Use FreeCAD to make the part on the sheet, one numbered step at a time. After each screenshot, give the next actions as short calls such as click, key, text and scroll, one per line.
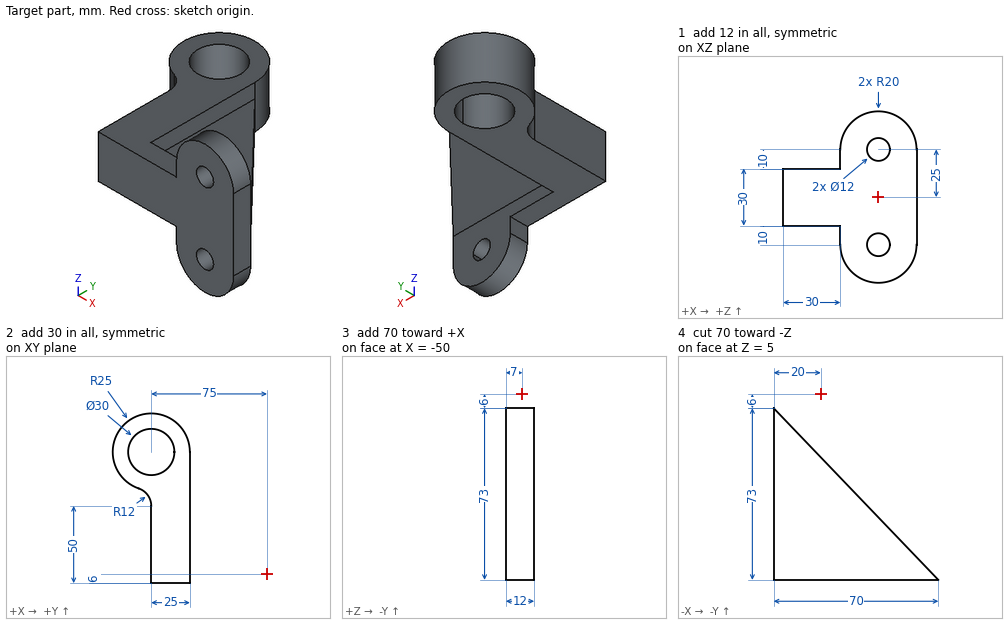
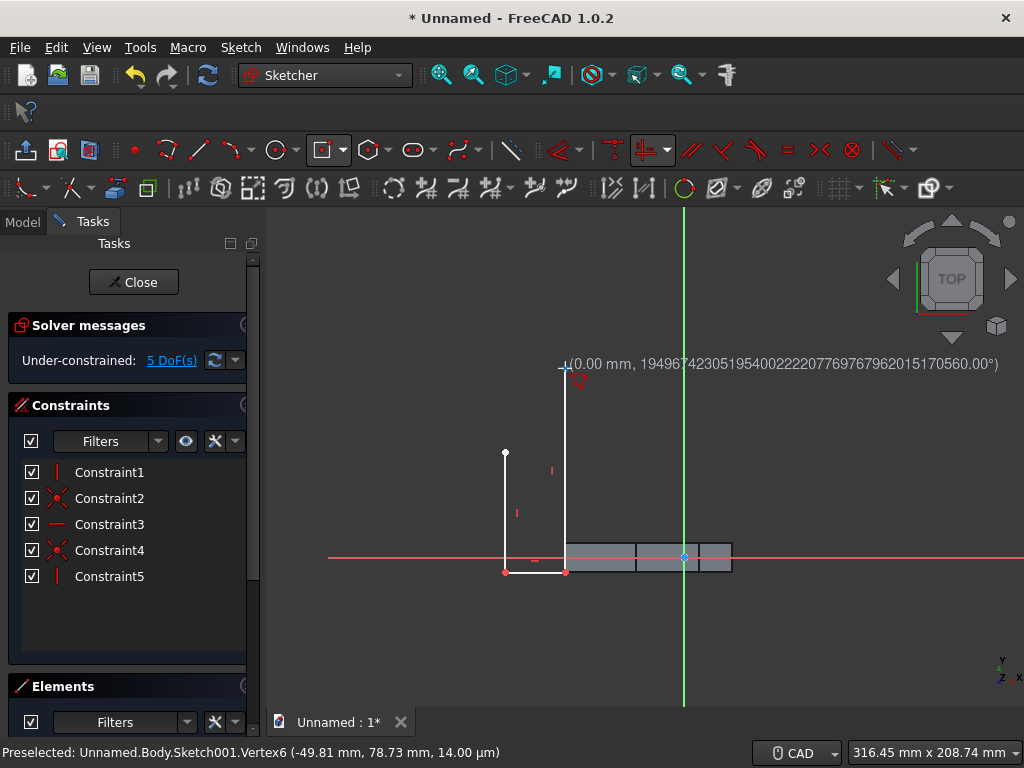
click(232, 150)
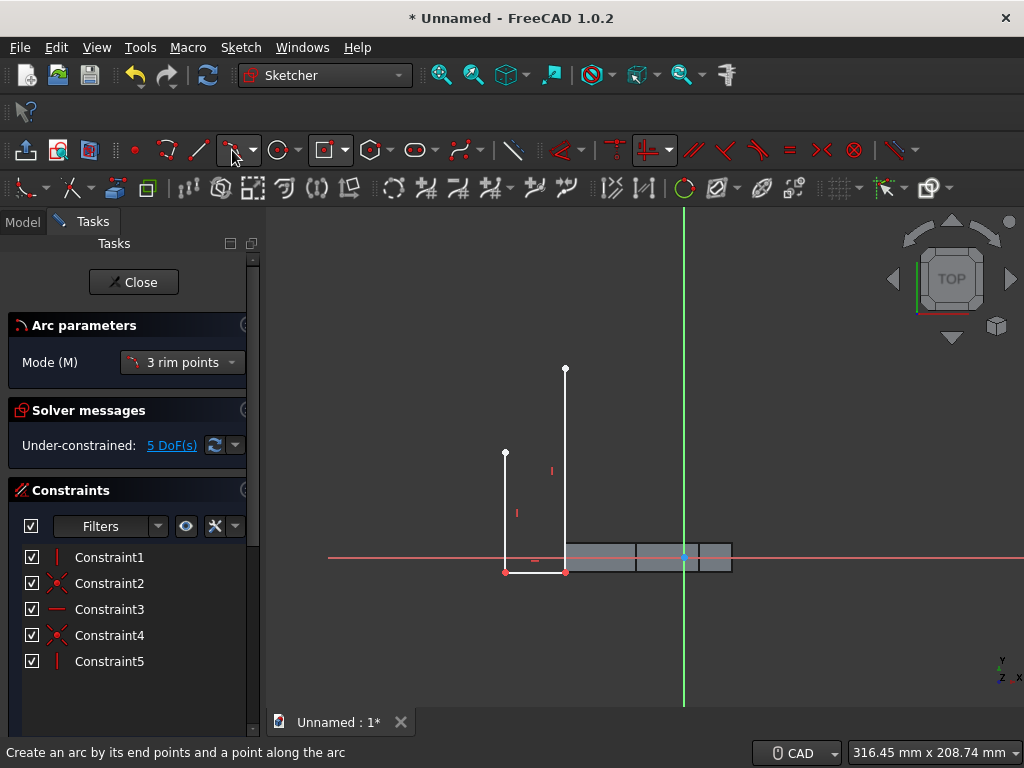
click(565, 369)
click(485, 425)
click(470, 320)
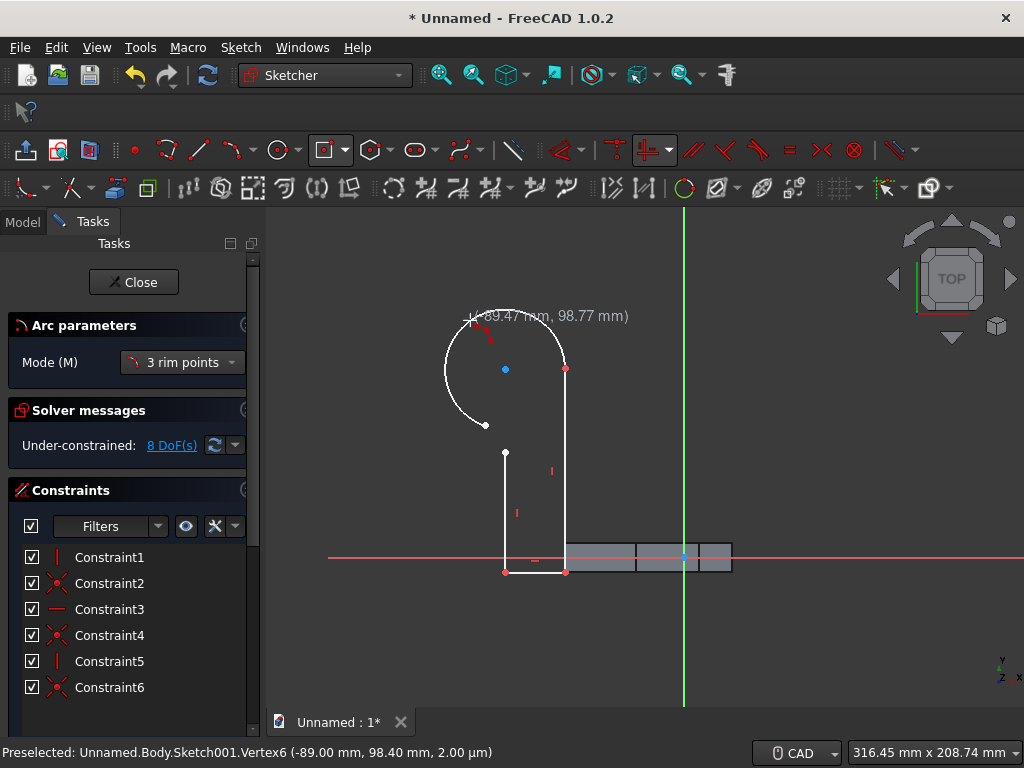
click(485, 426)
click(505, 453)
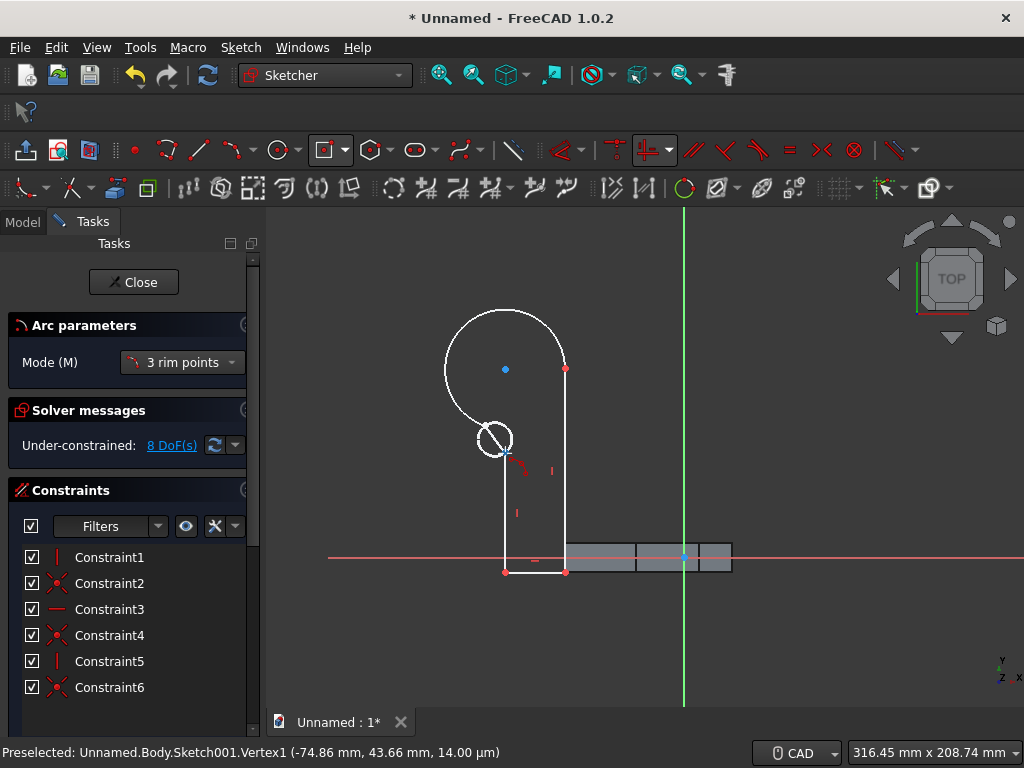
scroll(499, 435, up, 6)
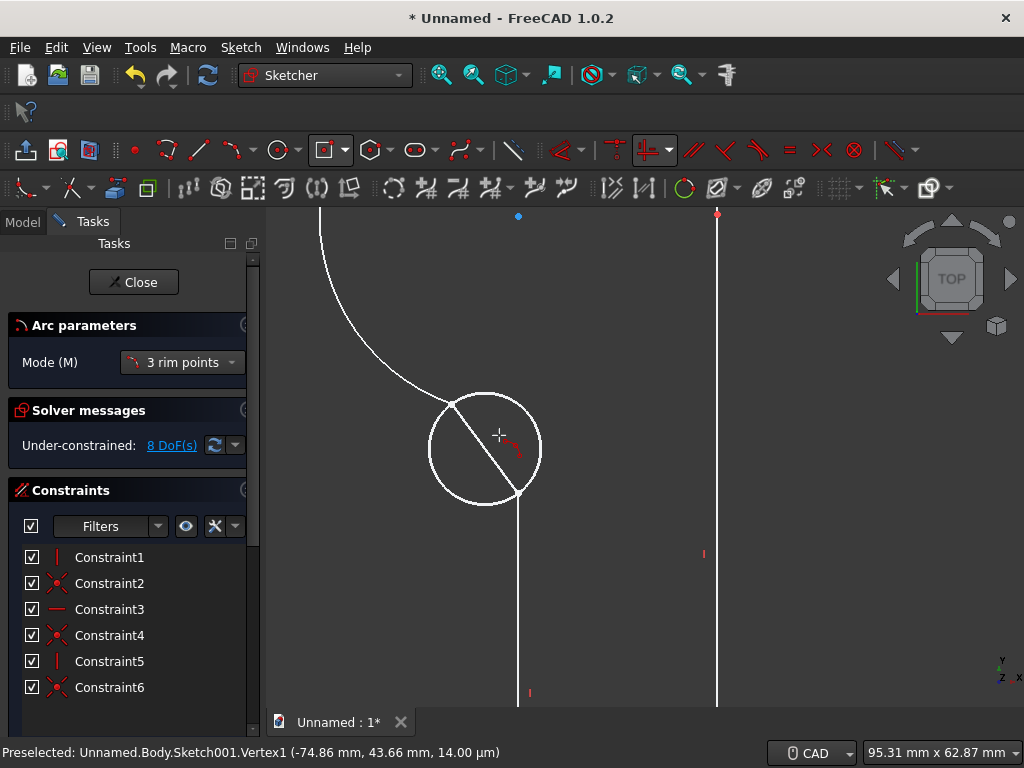
click(499, 436)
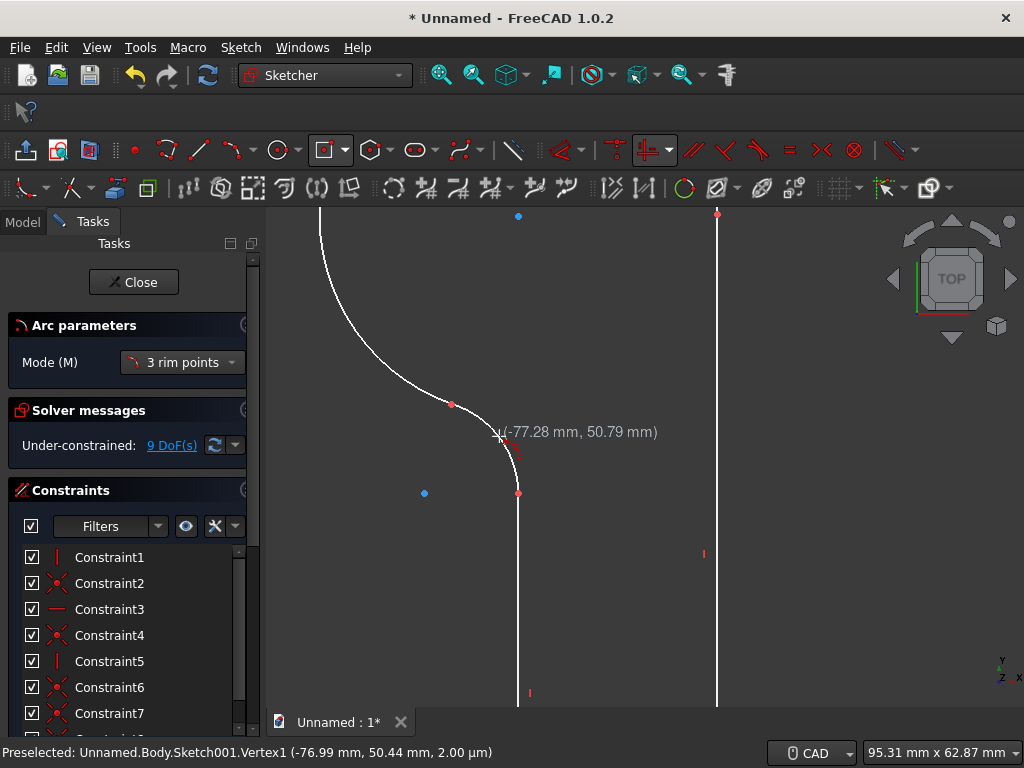
click(278, 150)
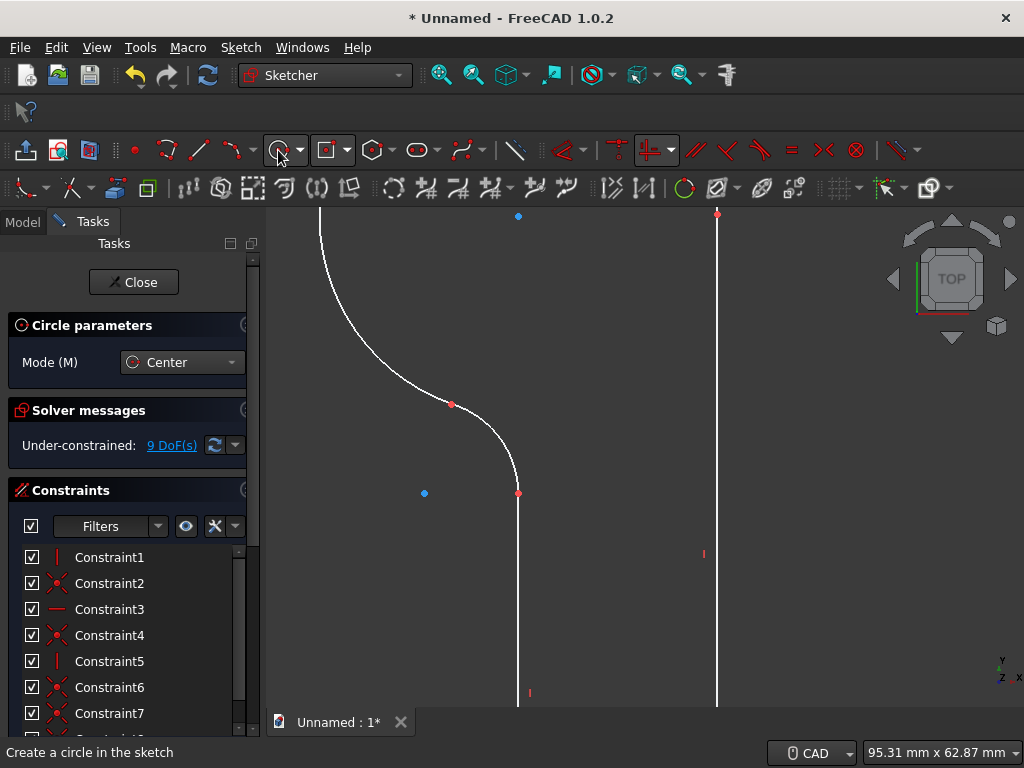
scroll(472, 450, down, 5)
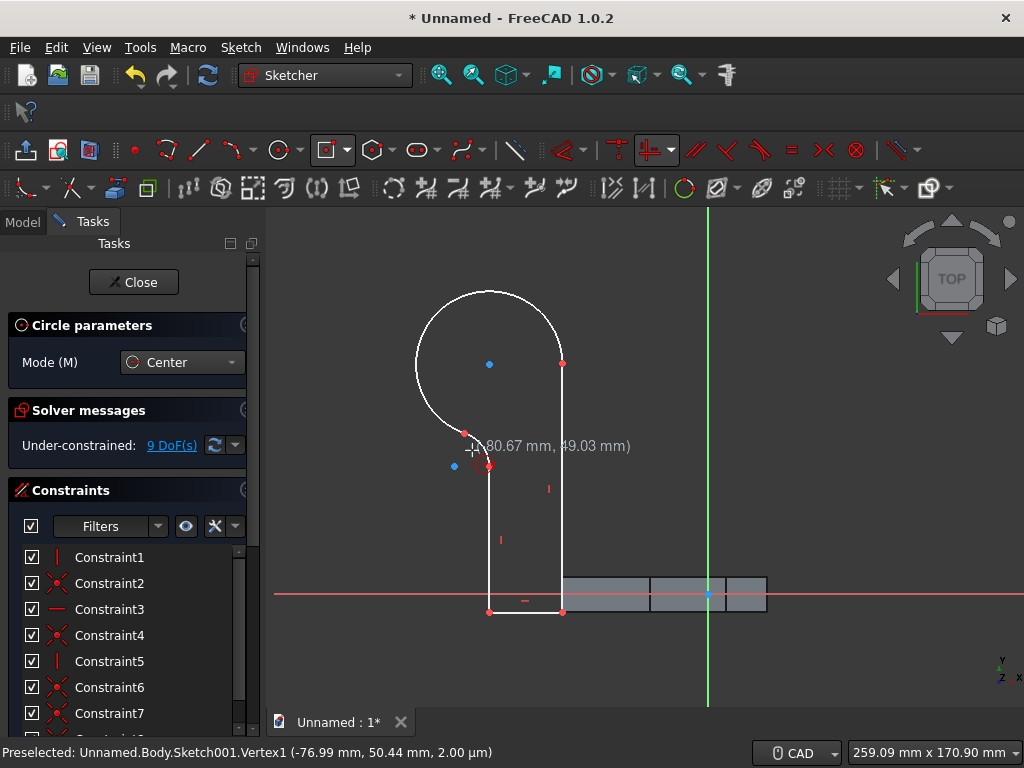
click(489, 363)
click(520, 332)
key(Escape)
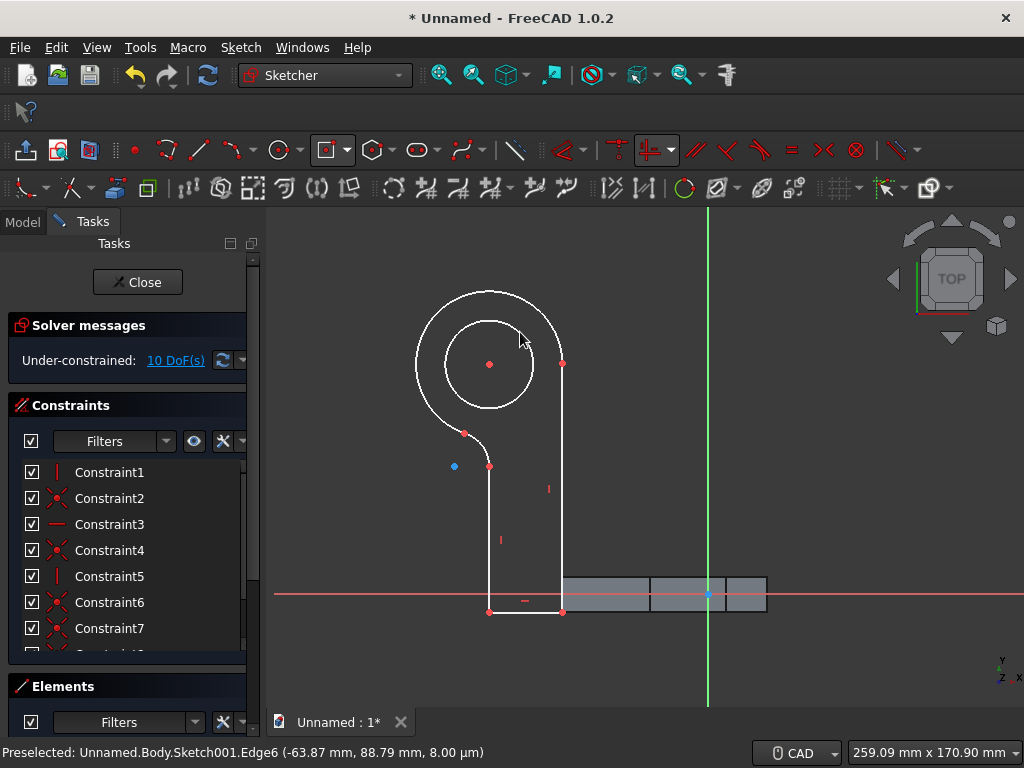
click(489, 510)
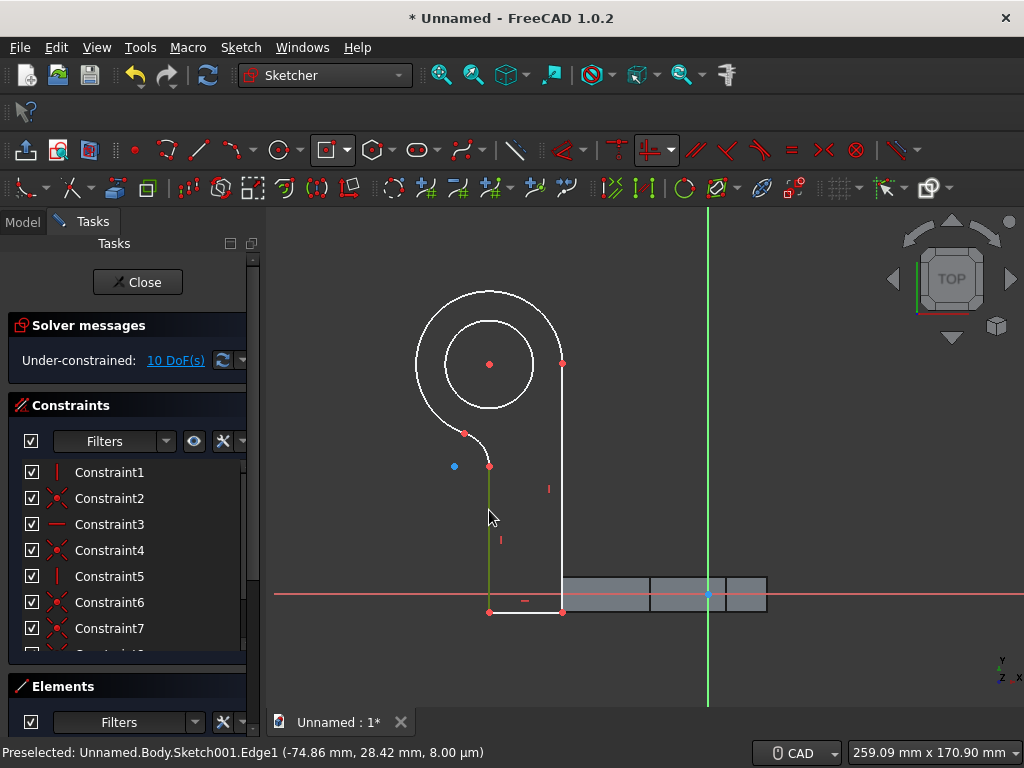
click(487, 454)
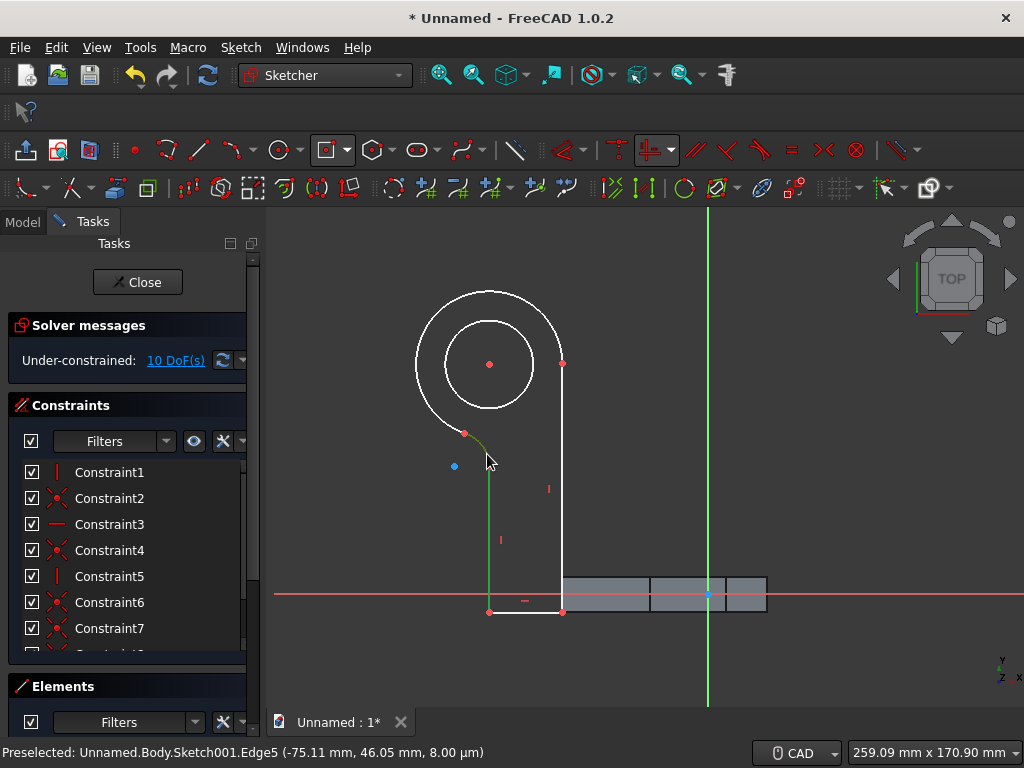
click(760, 150)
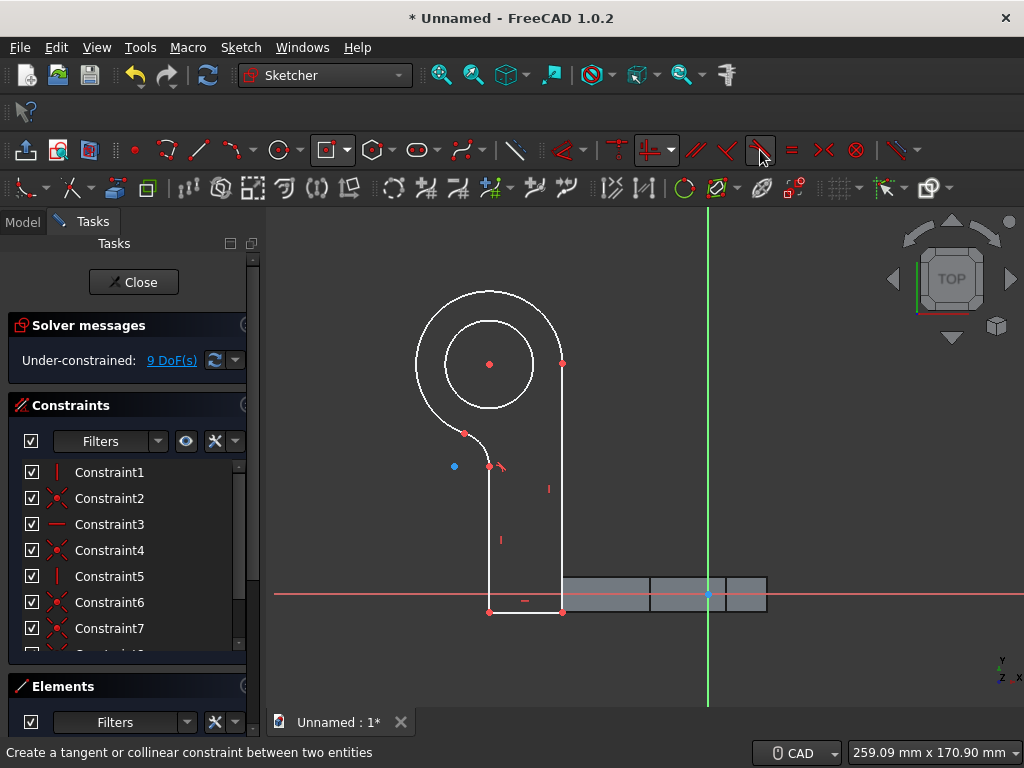
click(562, 538)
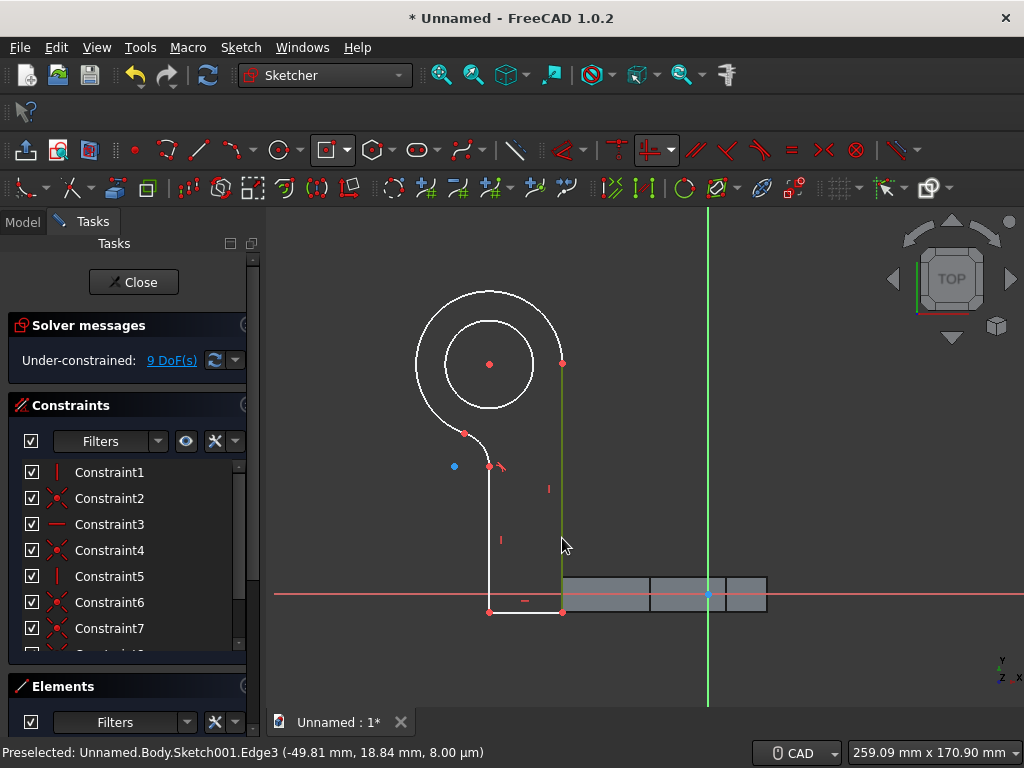
click(508, 294)